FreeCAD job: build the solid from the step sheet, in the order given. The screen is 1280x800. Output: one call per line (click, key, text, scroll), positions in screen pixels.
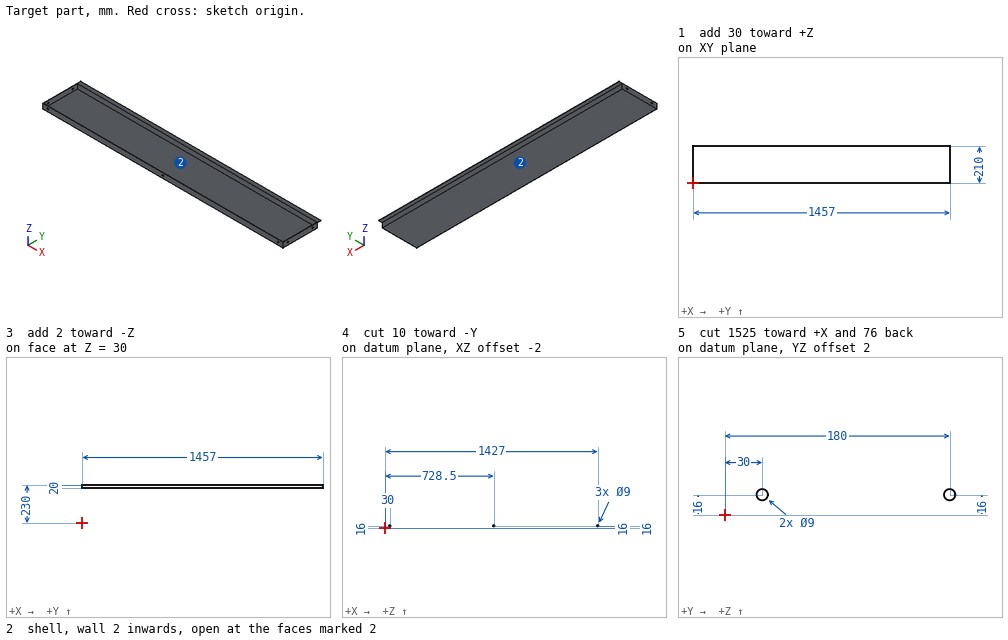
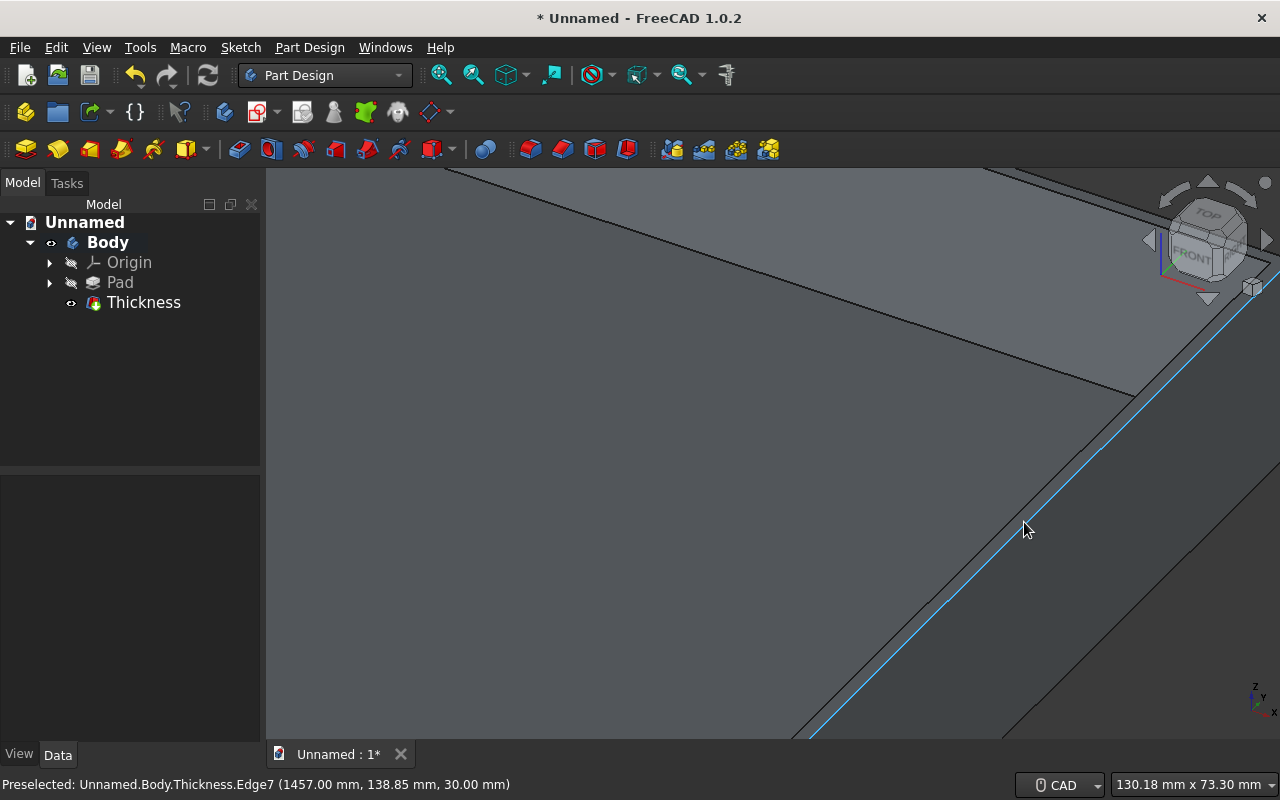
scroll(1012, 531, up, 5)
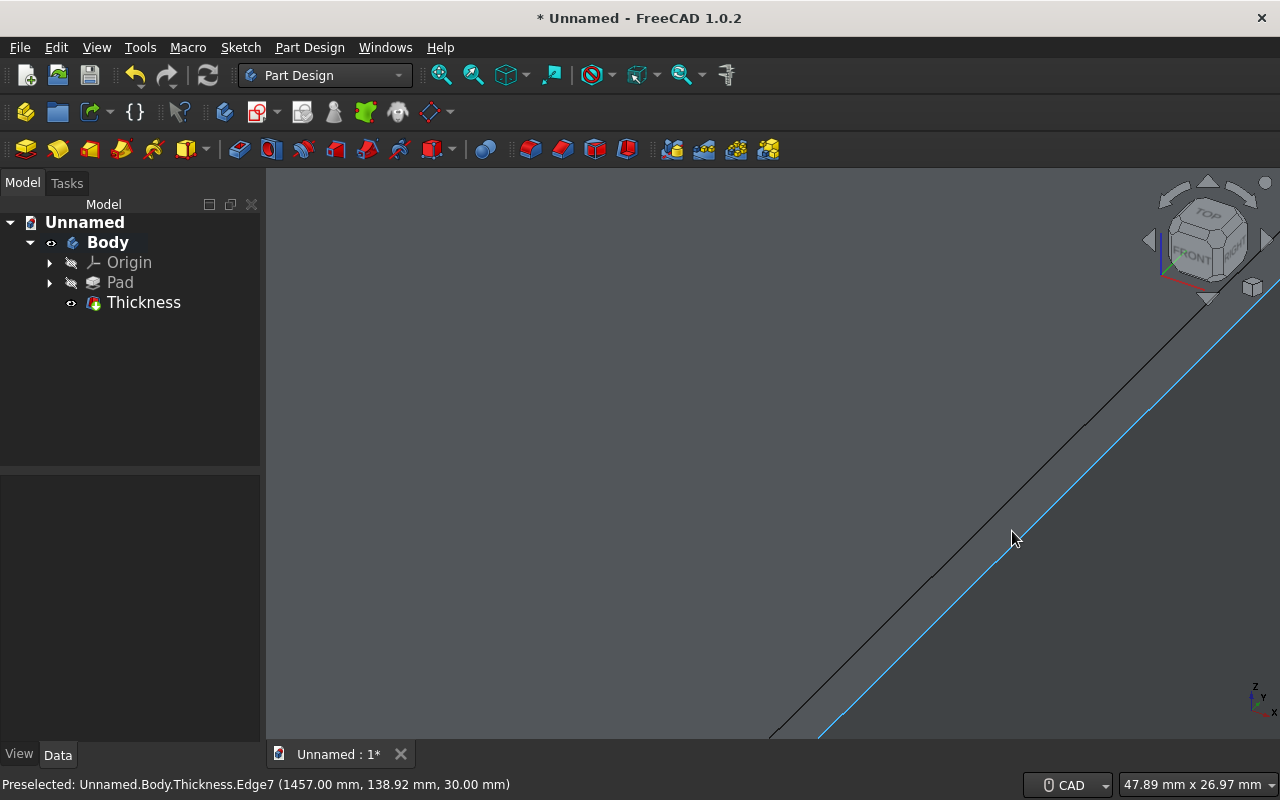
click(1010, 531)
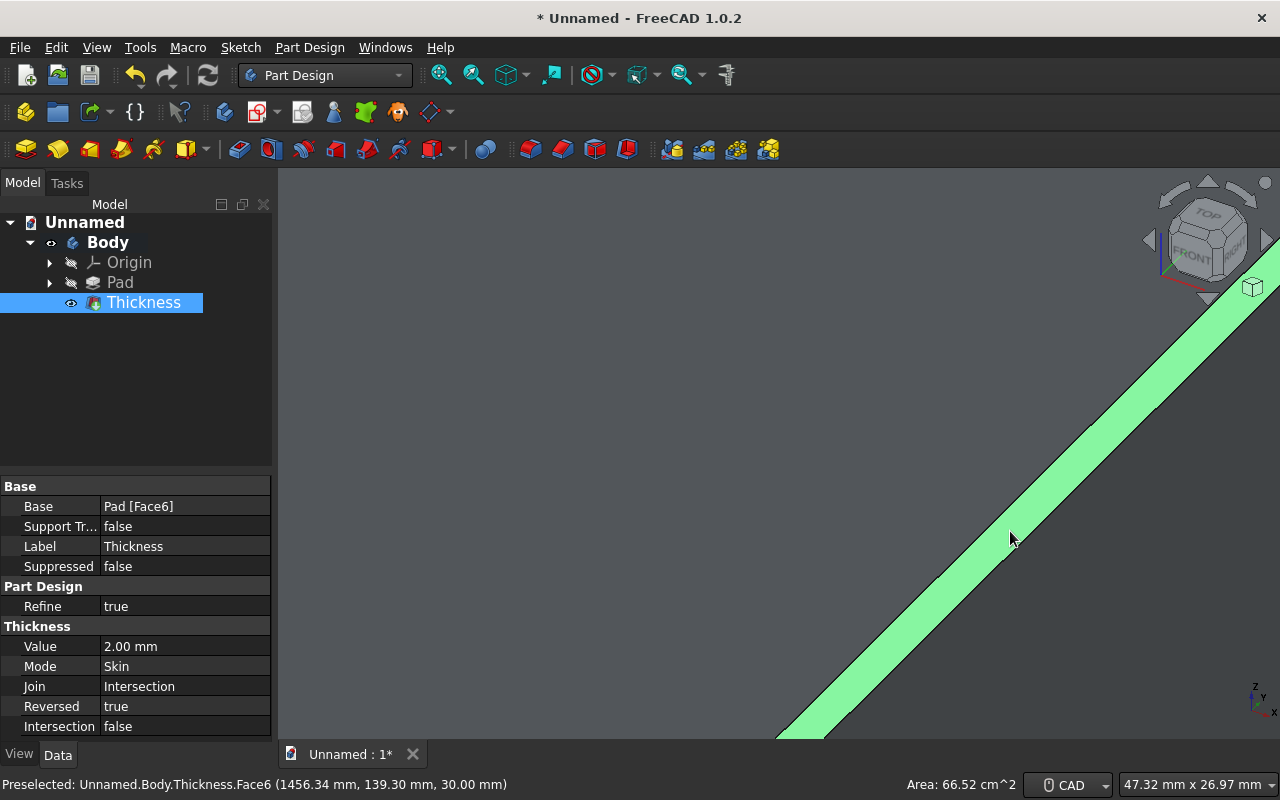
click(258, 112)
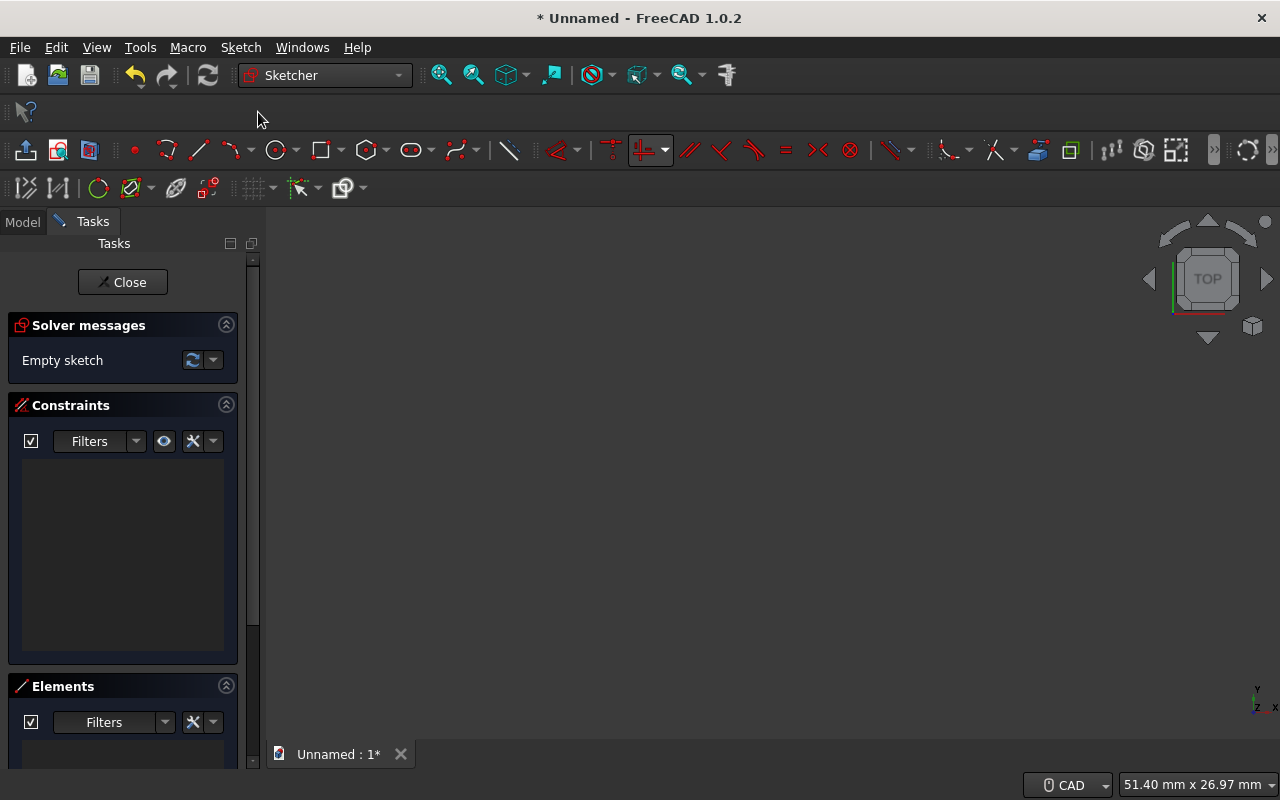
scroll(704, 473, down, 15)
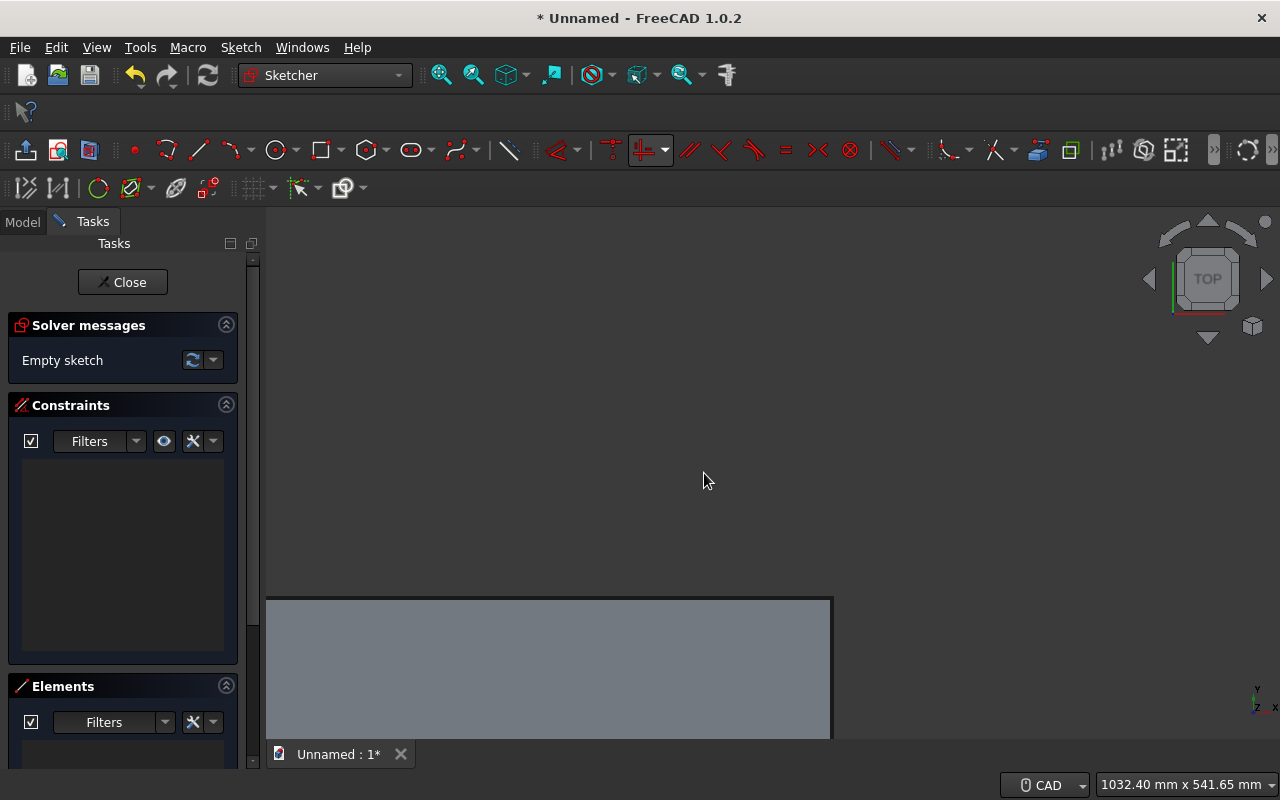
scroll(1046, 346, down, 5)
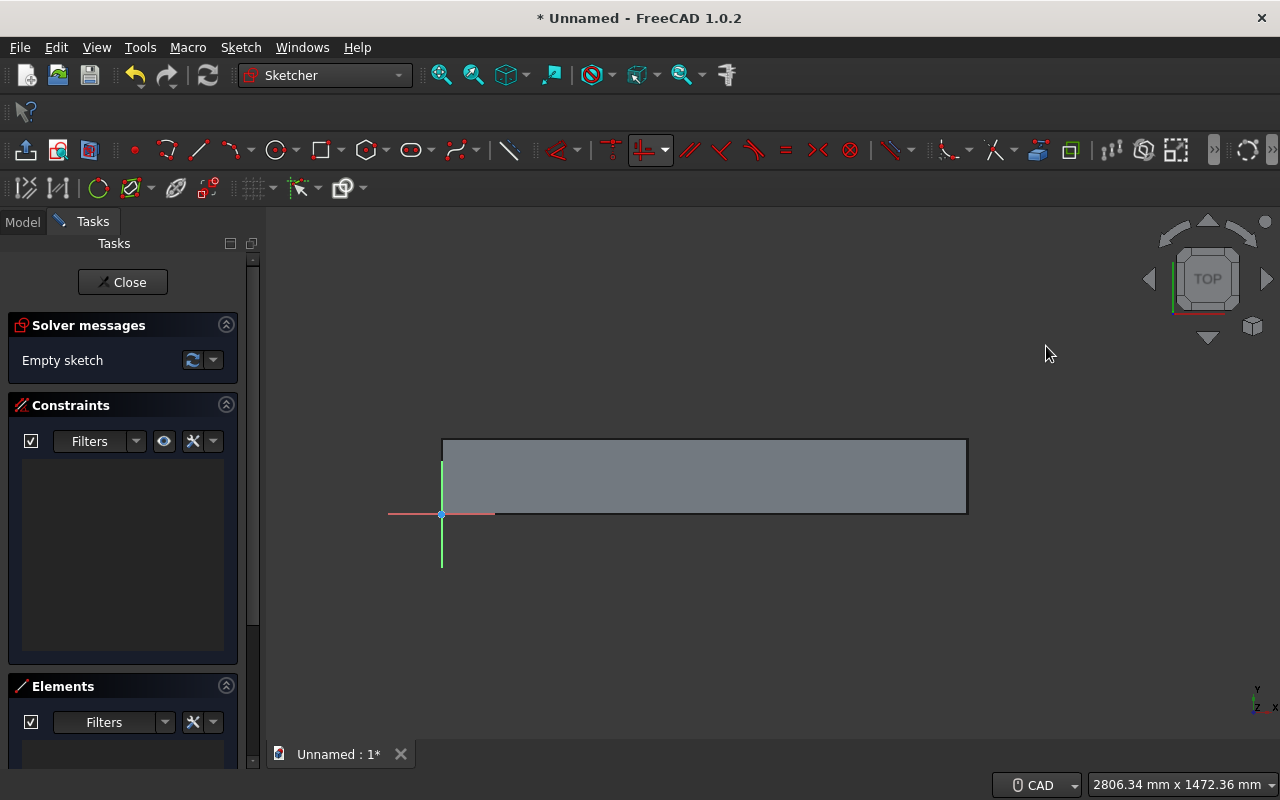
click(322, 150)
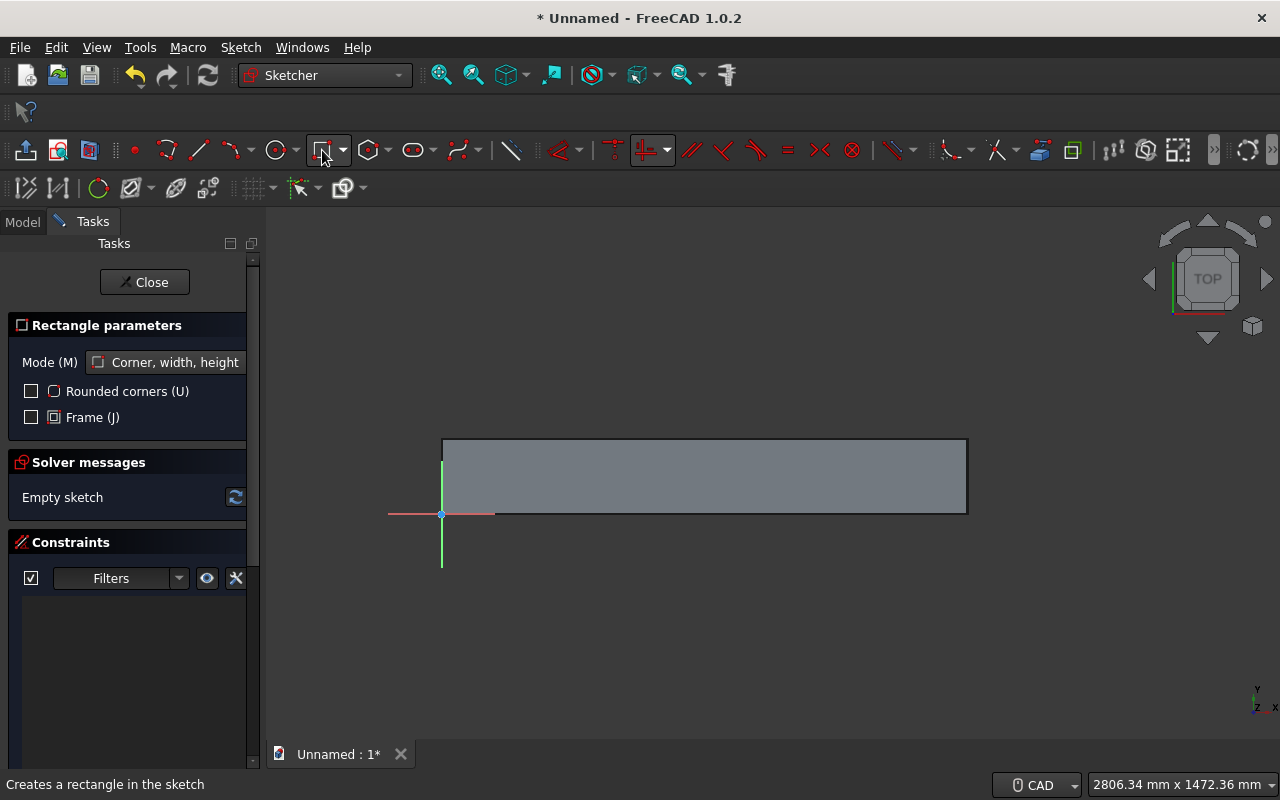
scroll(442, 431, up, 4)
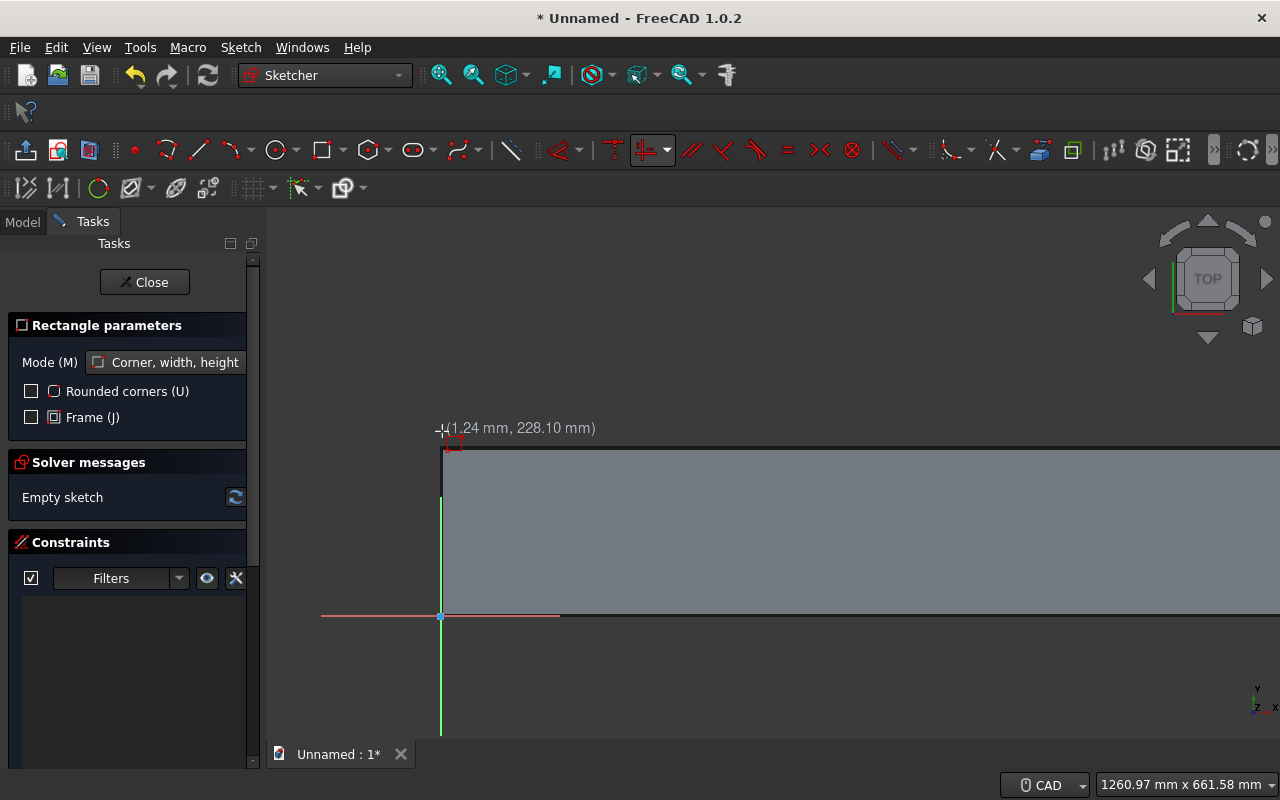
click(441, 431)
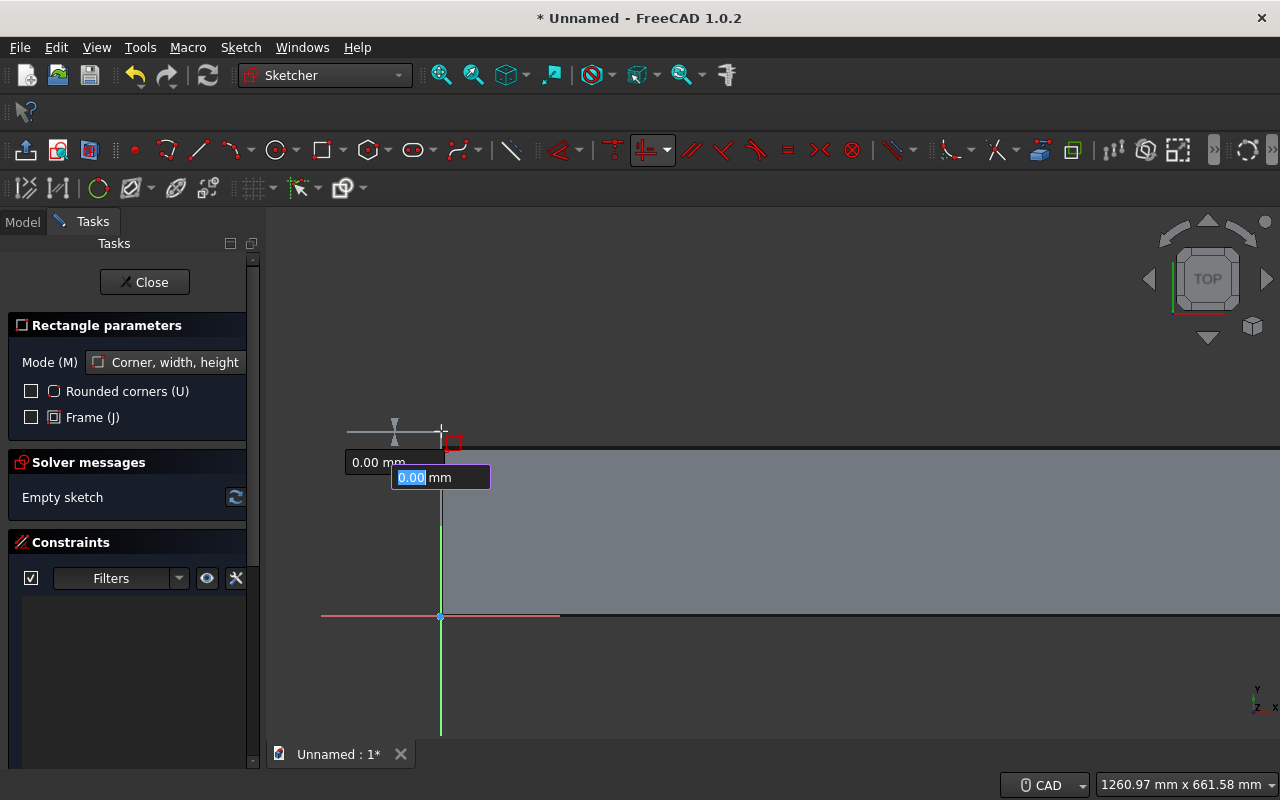
scroll(442, 432, down, 4)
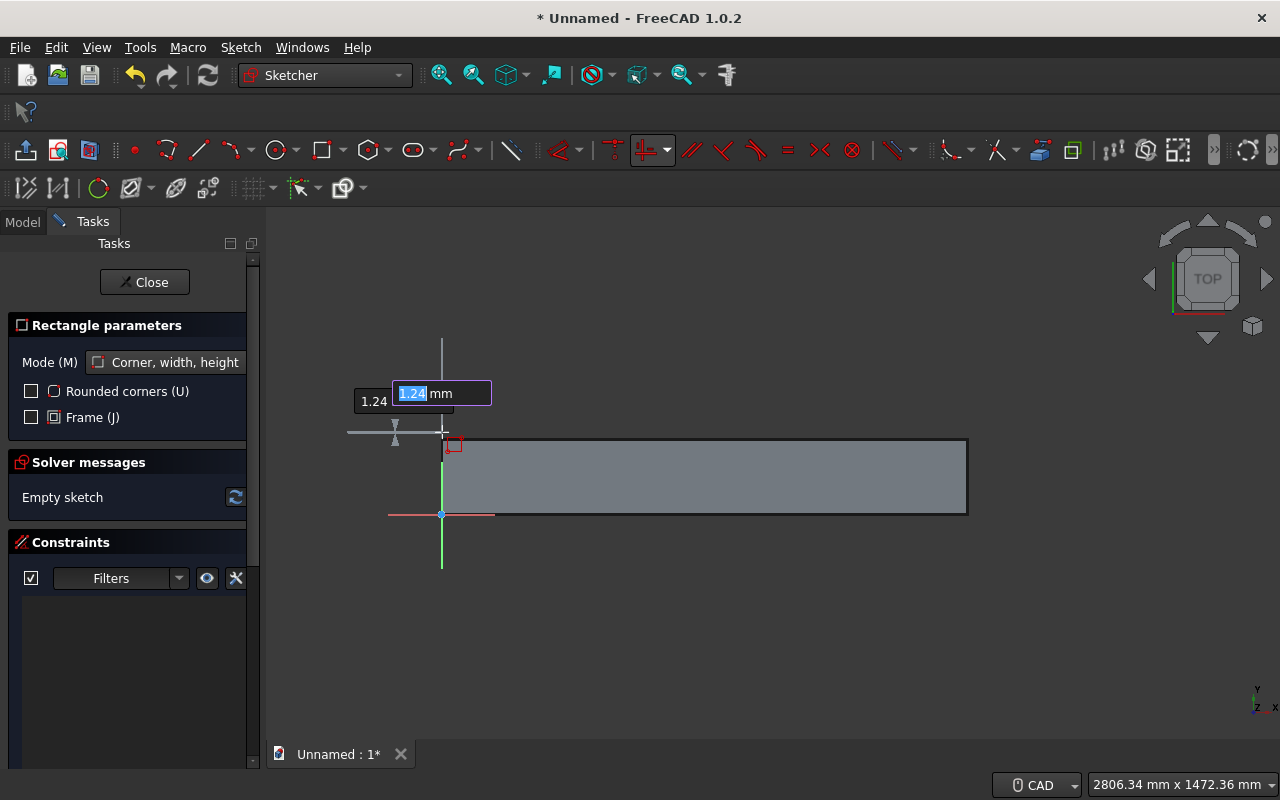
click(968, 439)
key(Escape)